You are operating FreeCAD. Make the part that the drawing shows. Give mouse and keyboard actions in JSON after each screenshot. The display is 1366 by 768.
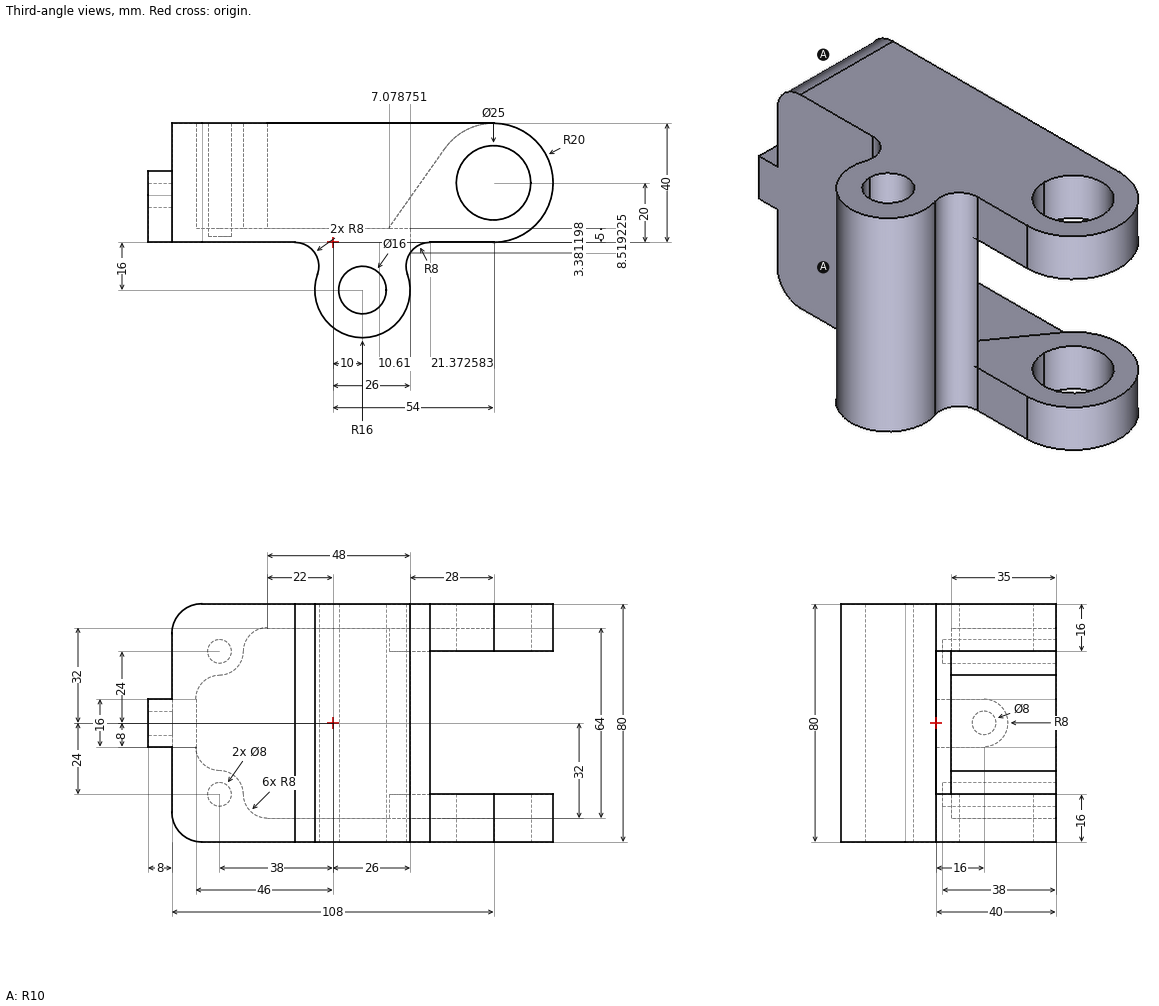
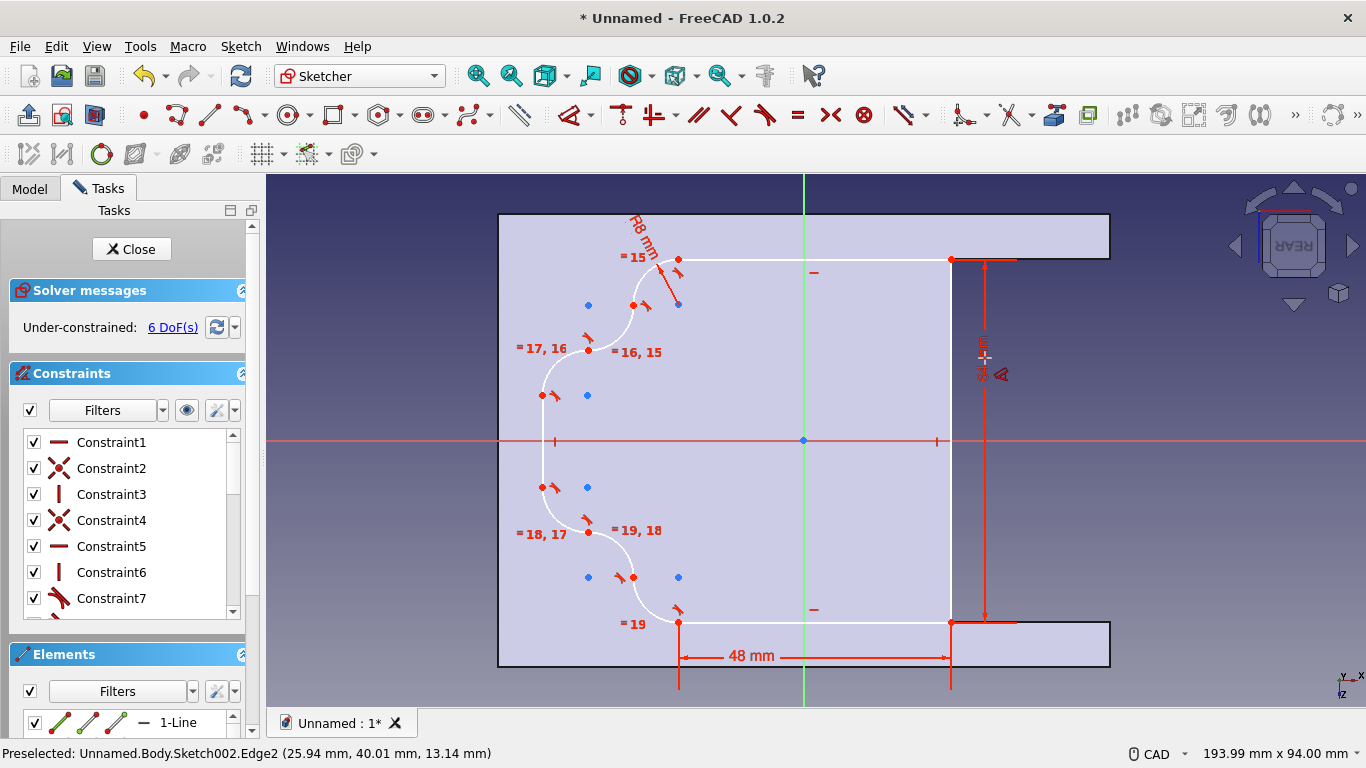
{"action": "left_click", "coordinate": [869, 260]}
{"action": "left_click", "coordinate": [752, 226]}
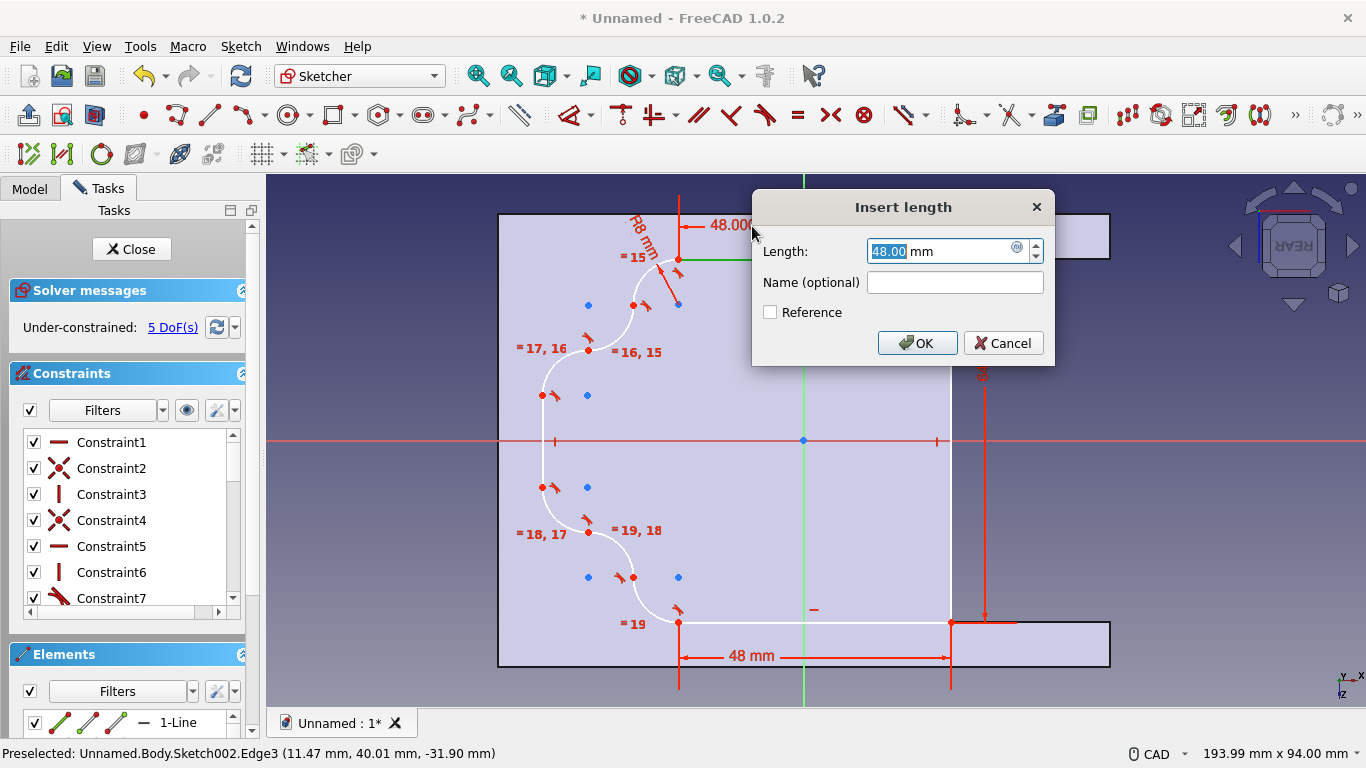
{"action": "type", "text": "48"}
{"action": "key", "text": "Return"}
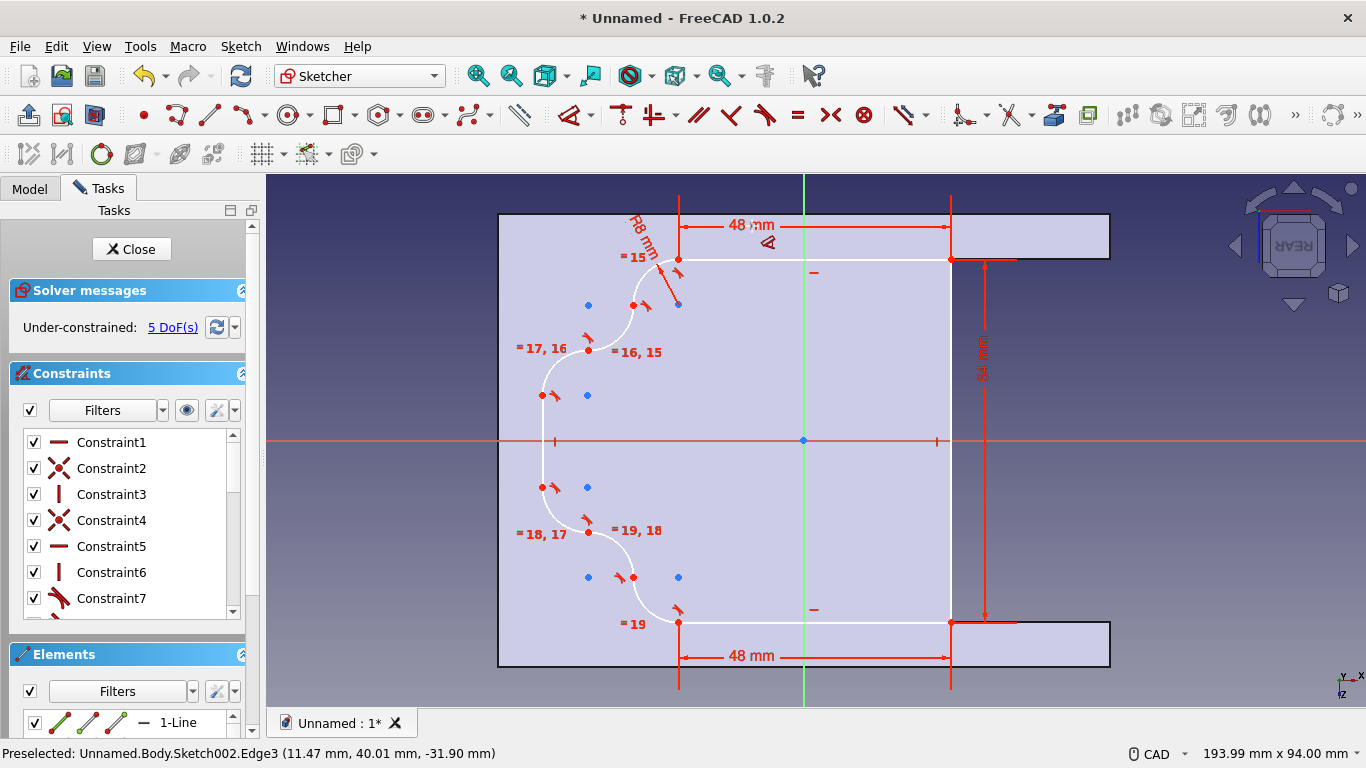
{"action": "left_click", "coordinate": [543, 423]}
{"action": "left_click", "coordinate": [509, 421]}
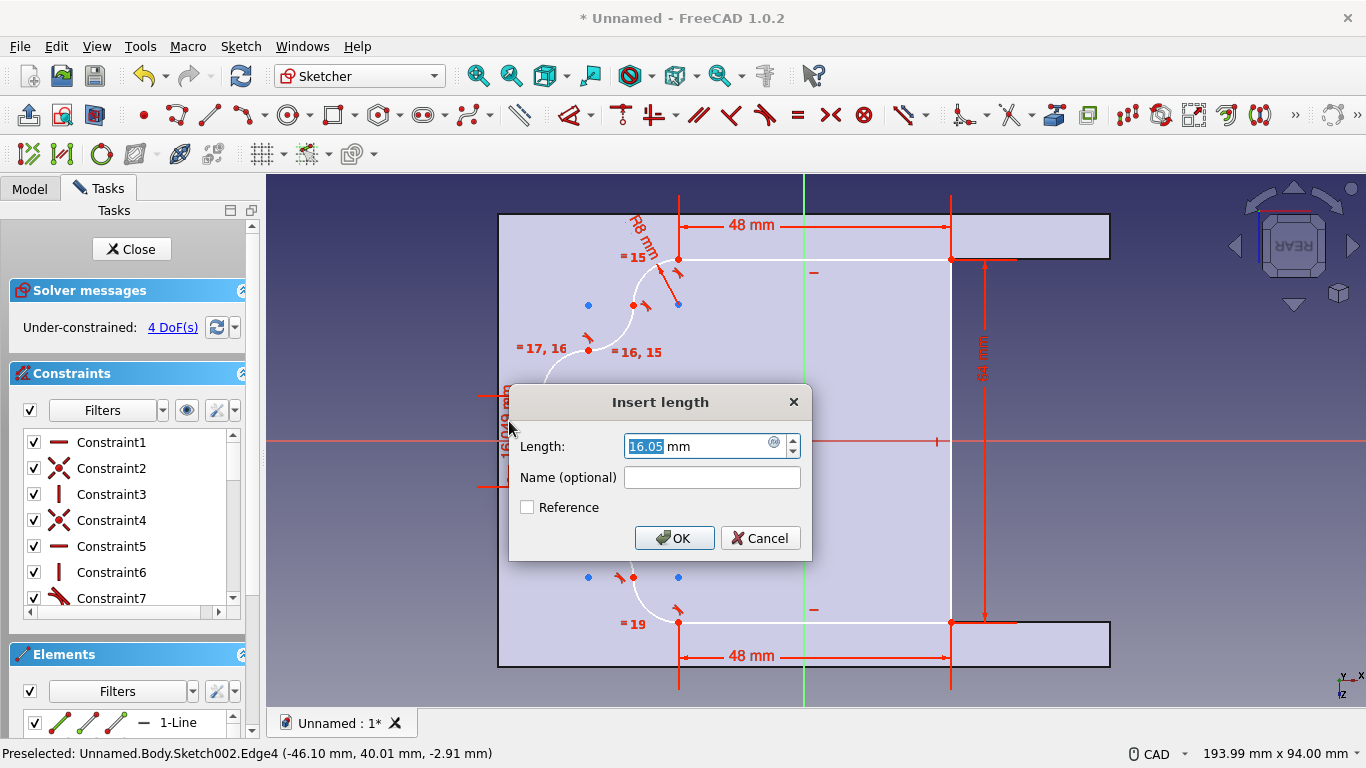
{"action": "type", "text": "16"}
{"action": "key", "text": "Return"}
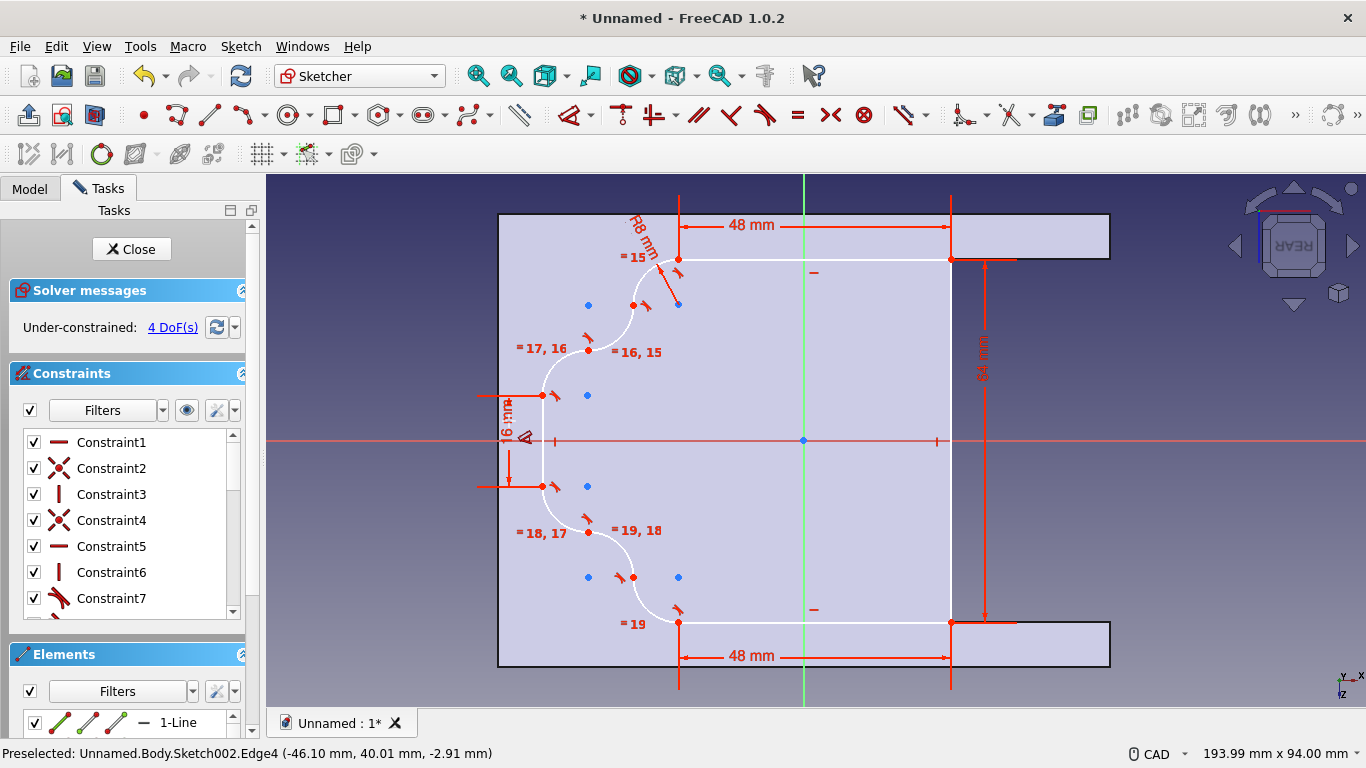
{"action": "left_click", "coordinate": [543, 396]}
{"action": "left_click", "coordinate": [838, 418]}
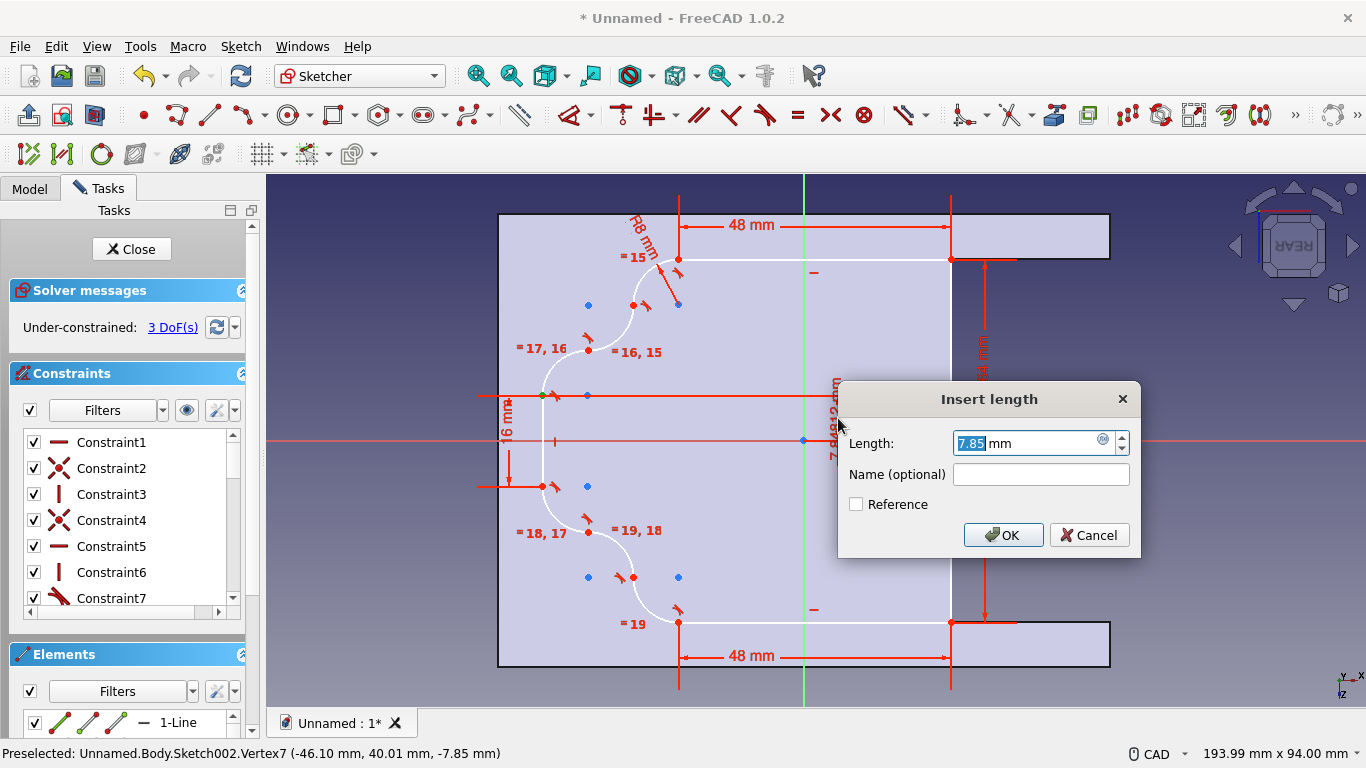
{"action": "type", "text": "8"}
{"action": "key", "text": "Return"}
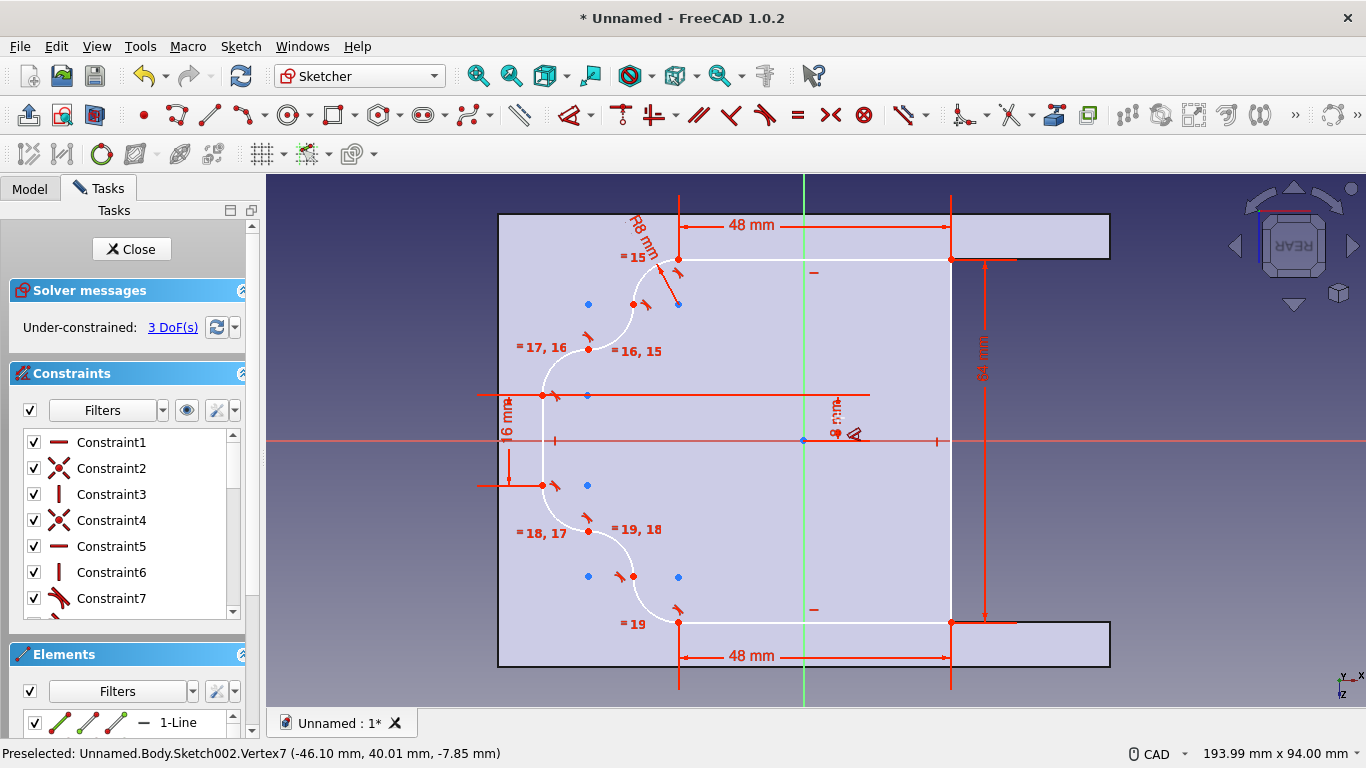
{"action": "left_click", "coordinate": [679, 623]}
{"action": "left_click", "coordinate": [741, 406]}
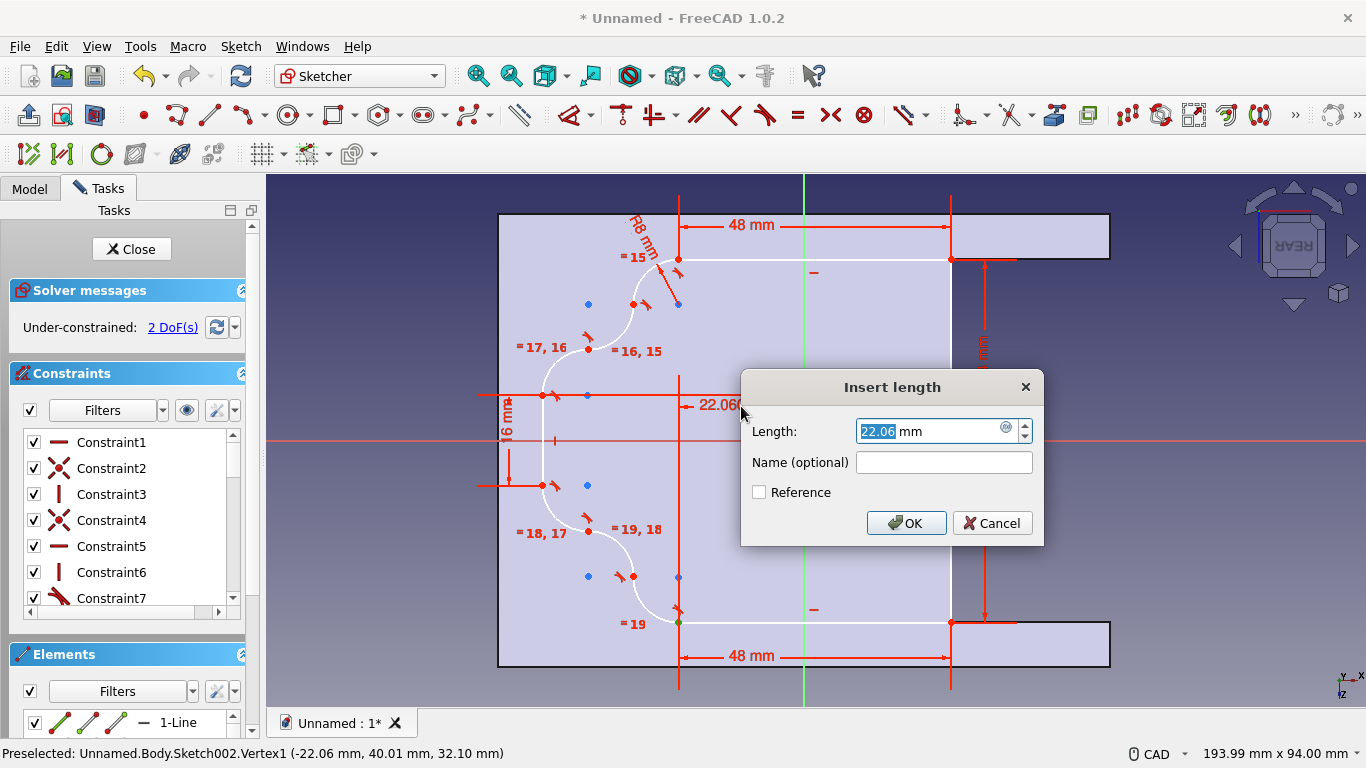
{"action": "type", "text": "22"}
{"action": "key", "text": "Return"}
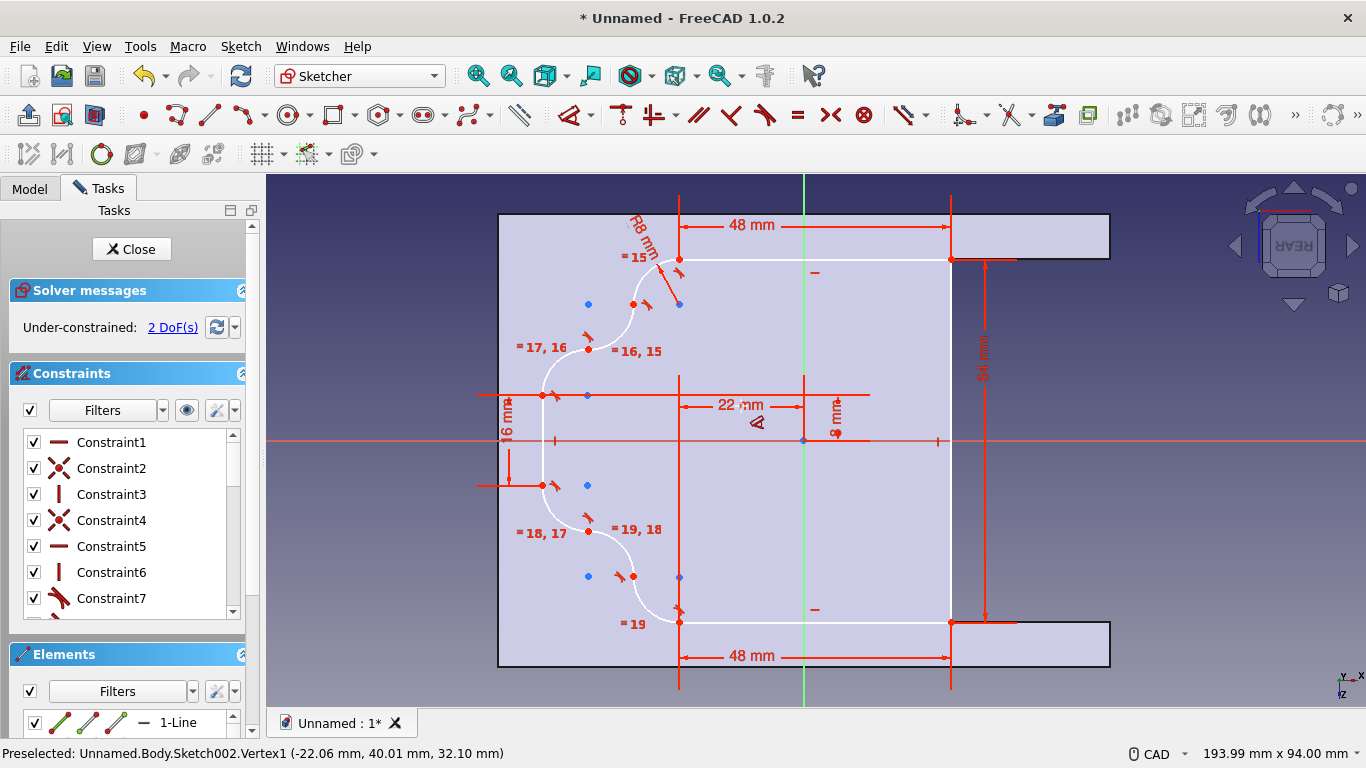
{"action": "left_click", "coordinate": [679, 623]}
{"action": "left_click", "coordinate": [645, 532]}